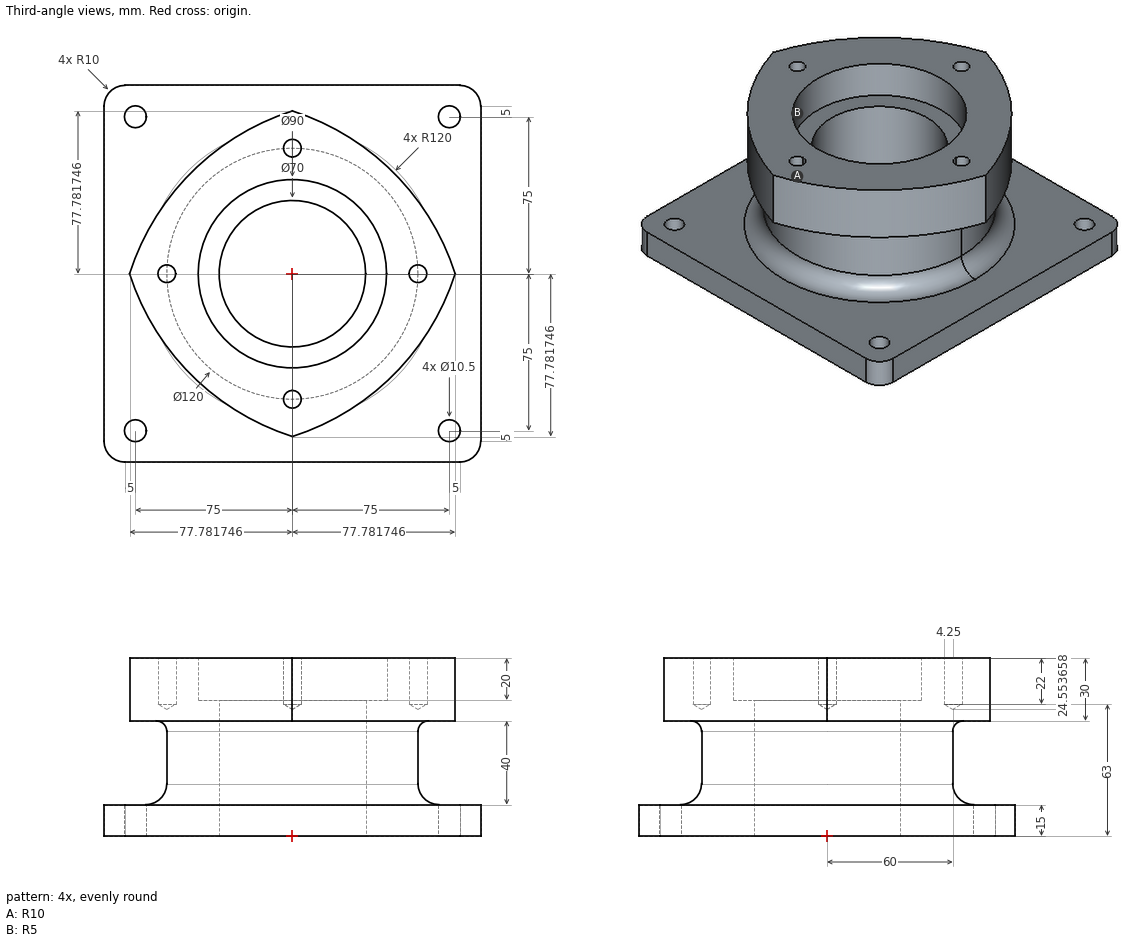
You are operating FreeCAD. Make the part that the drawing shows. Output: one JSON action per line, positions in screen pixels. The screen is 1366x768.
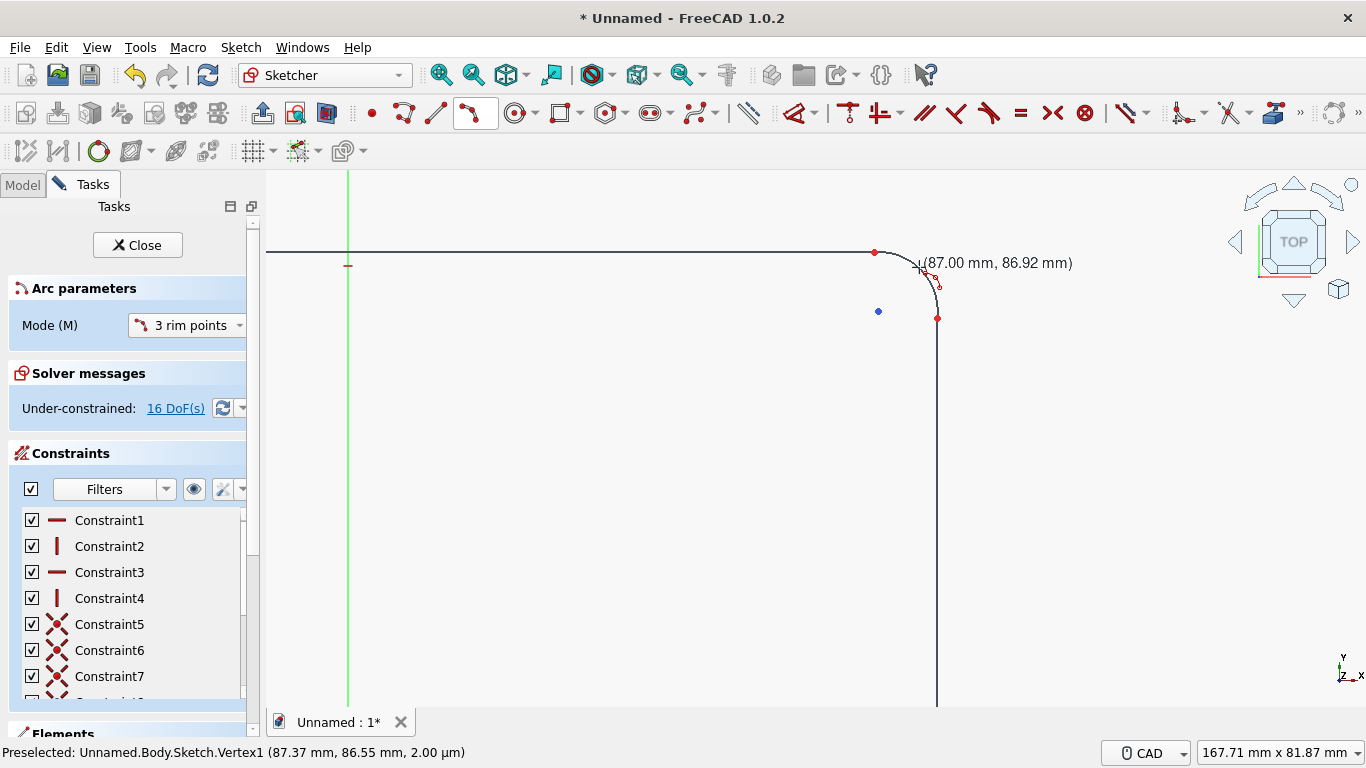
{"action": "left_click", "coordinate": [516, 114]}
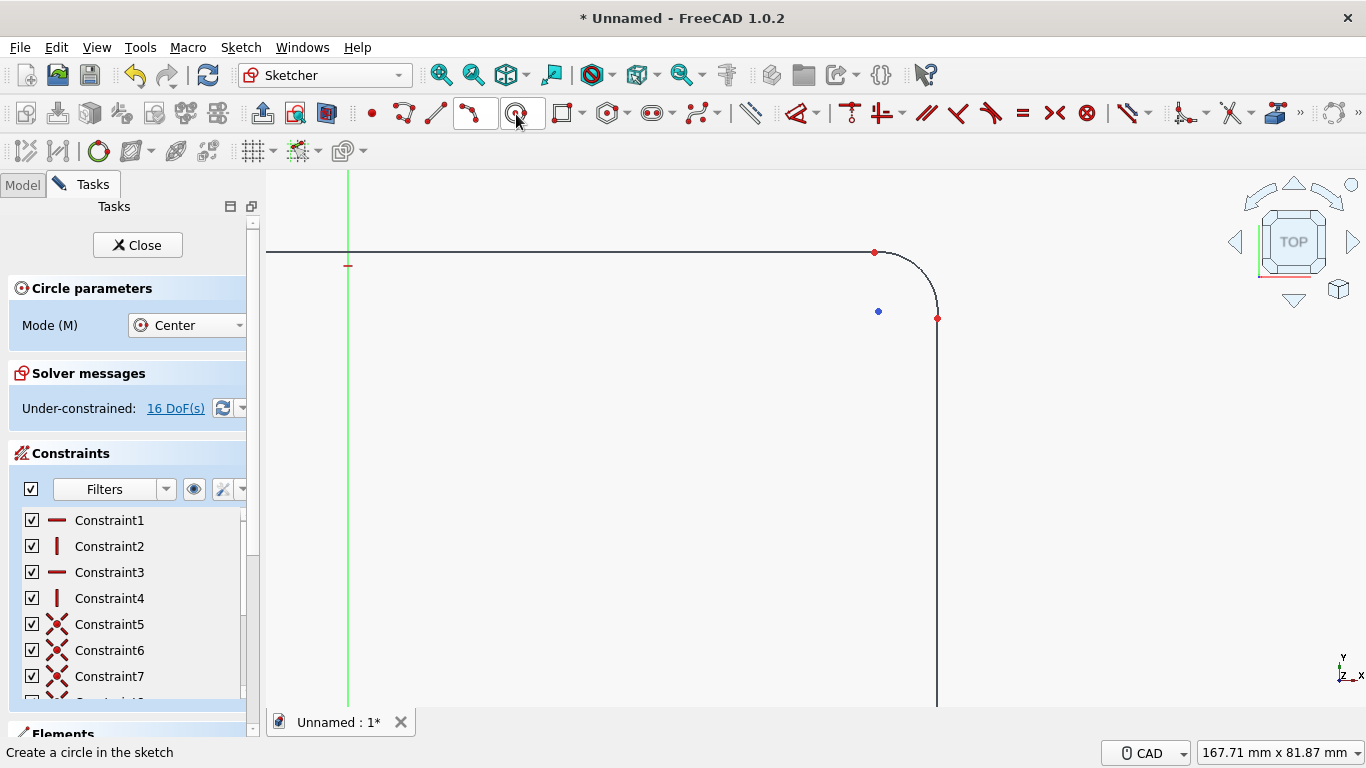
{"action": "scroll", "coordinate": [920, 266], "scroll_direction": "down", "scroll_amount": 6}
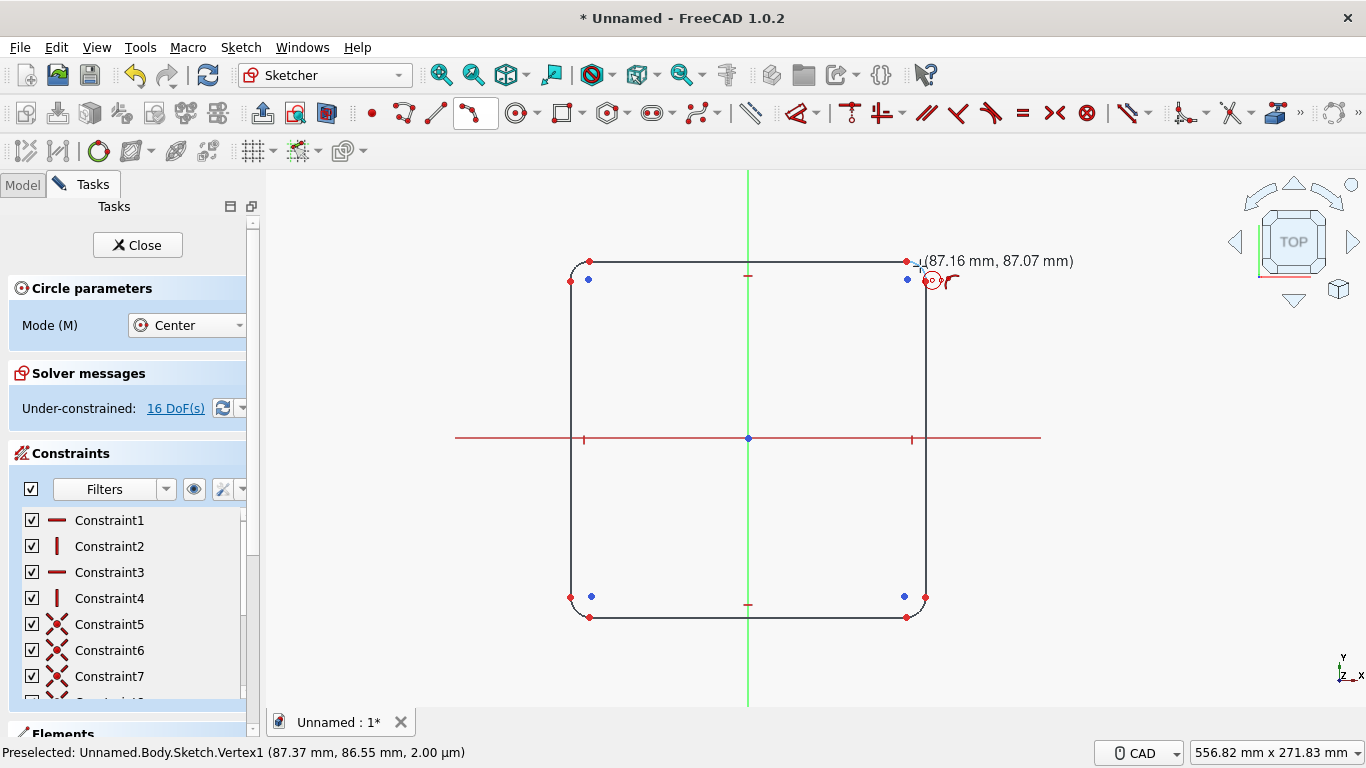
{"action": "scroll", "coordinate": [896, 587], "scroll_direction": "up", "scroll_amount": 4}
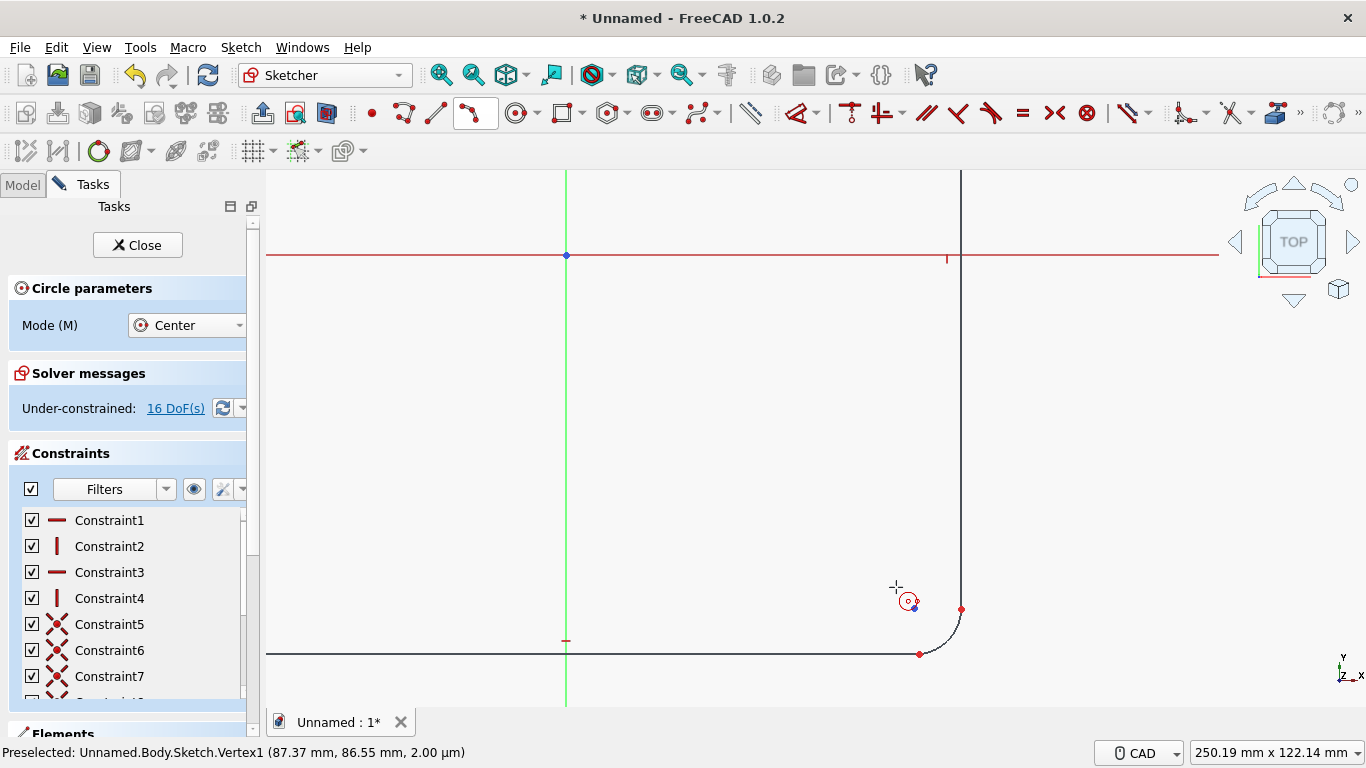
{"action": "left_click", "coordinate": [896, 585]}
{"action": "mouse_move", "coordinate": [913, 569]}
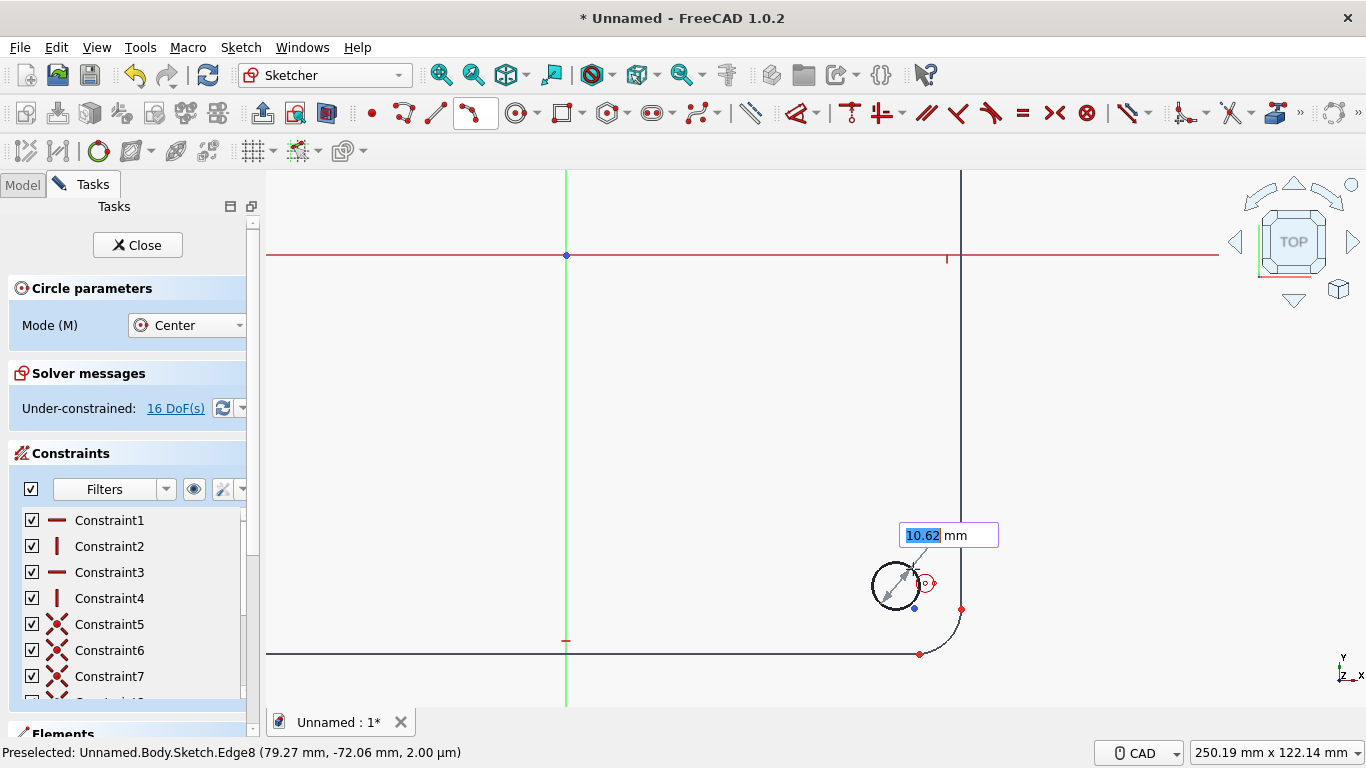
{"action": "type", "text": "10.5"}
{"action": "key", "text": "Return"}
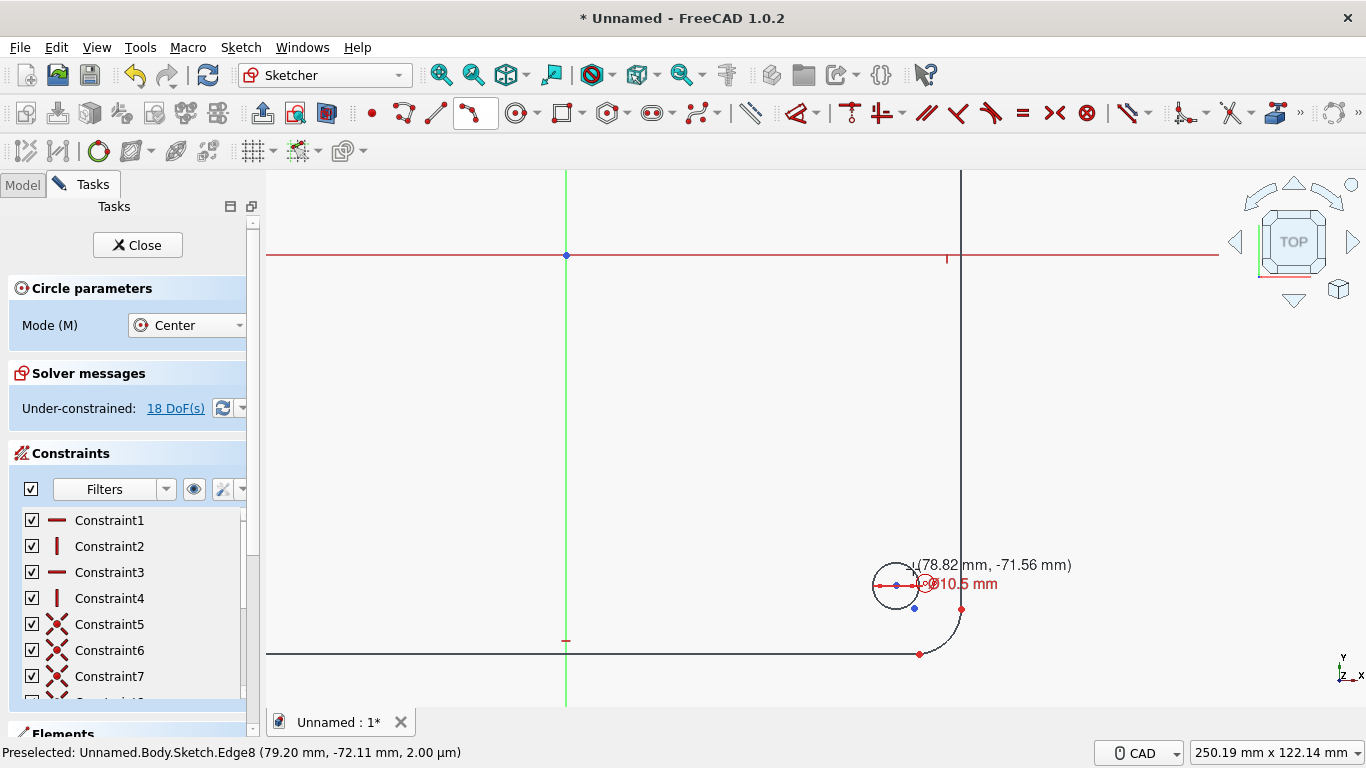
{"action": "scroll", "coordinate": [895, 588], "scroll_direction": "down", "scroll_amount": 4}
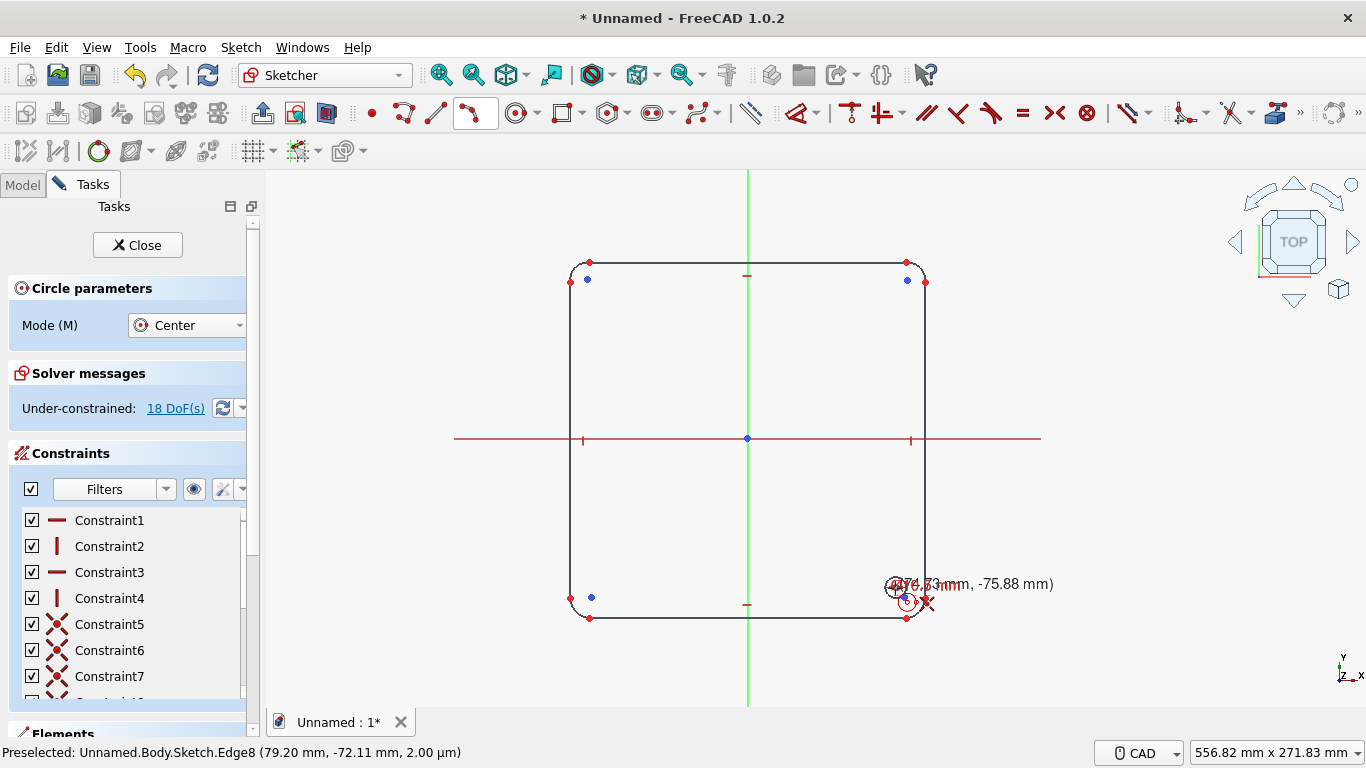
{"action": "scroll", "coordinate": [600, 587], "scroll_direction": "up", "scroll_amount": 4}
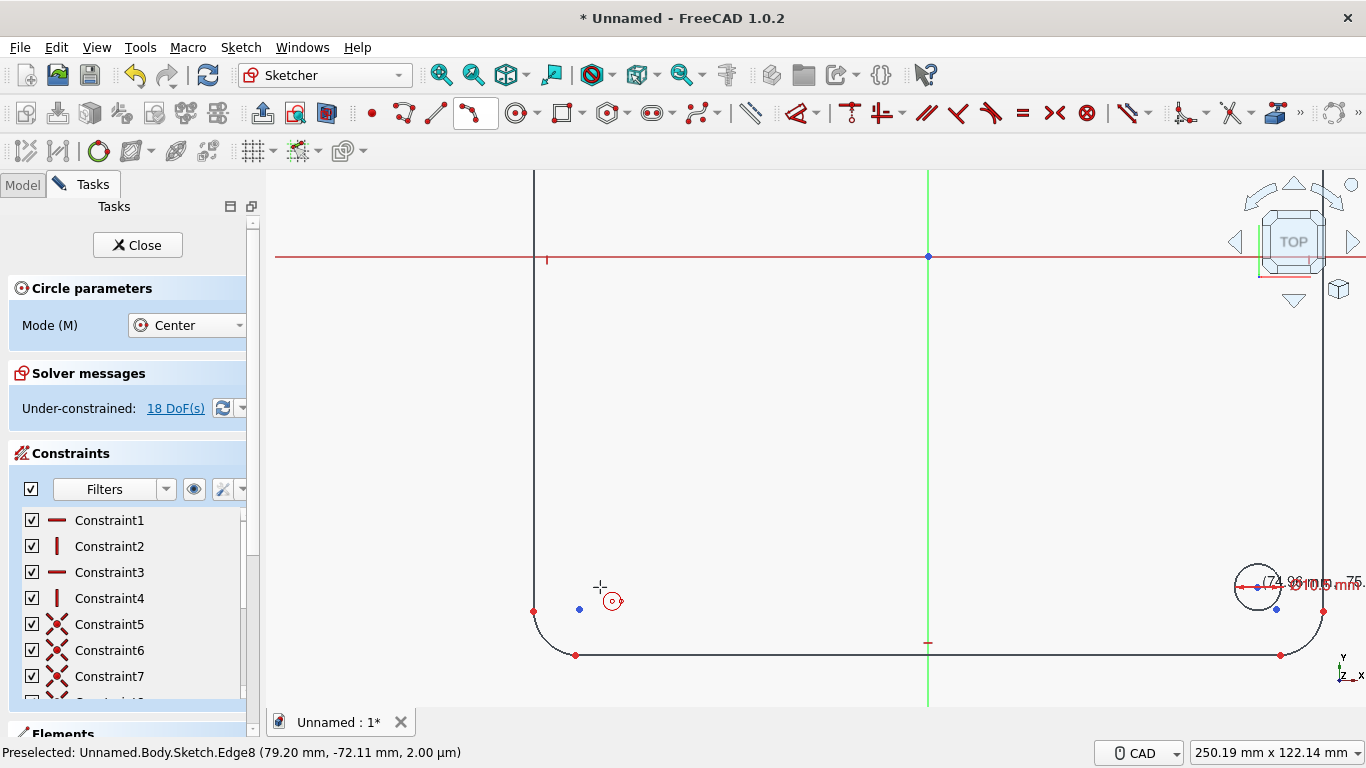
{"action": "left_click", "coordinate": [599, 586]}
{"action": "mouse_move", "coordinate": [615, 570]}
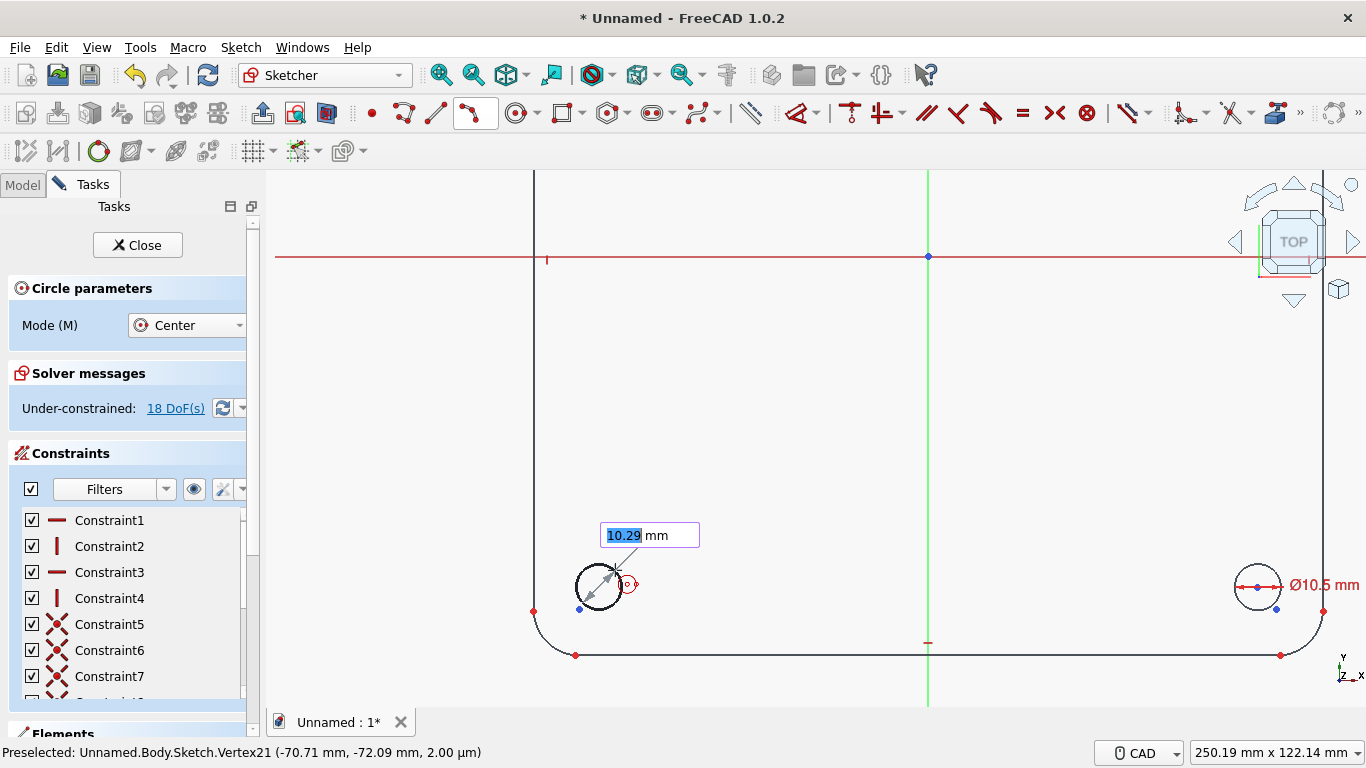
{"action": "type", "text": "10.5"}
{"action": "key", "text": "Return"}